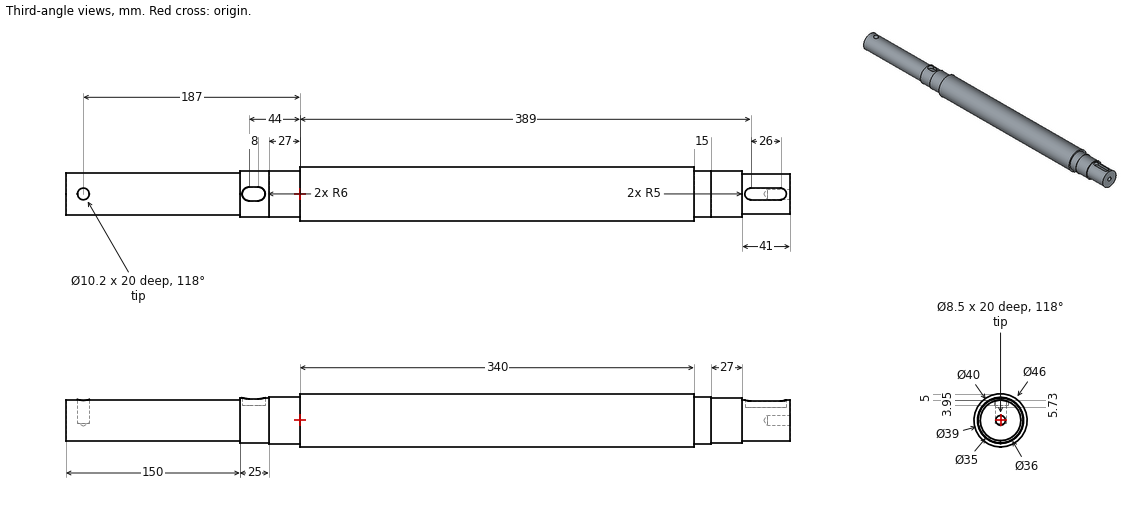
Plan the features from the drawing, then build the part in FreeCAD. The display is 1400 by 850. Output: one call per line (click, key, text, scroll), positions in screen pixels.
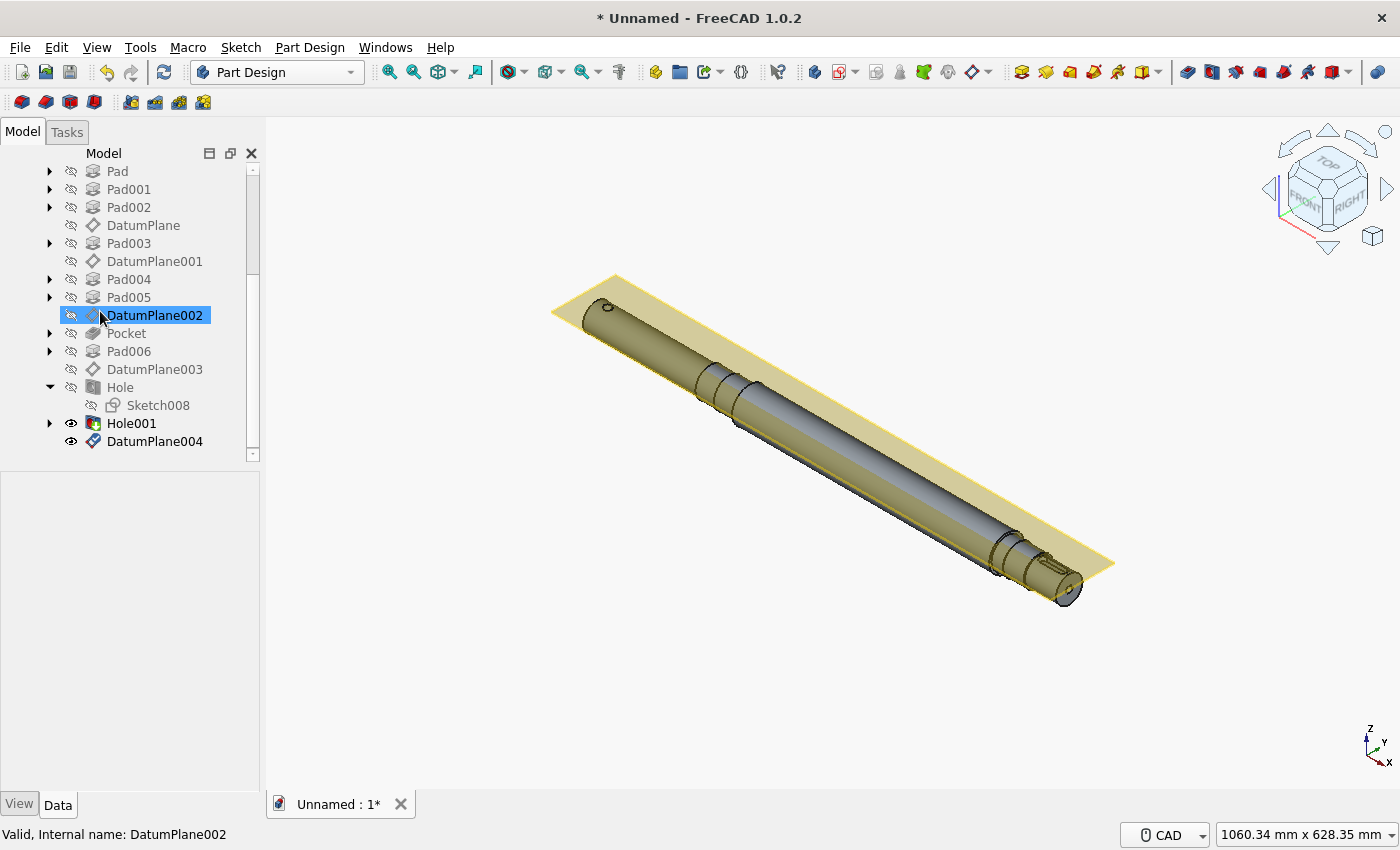
click(116, 441)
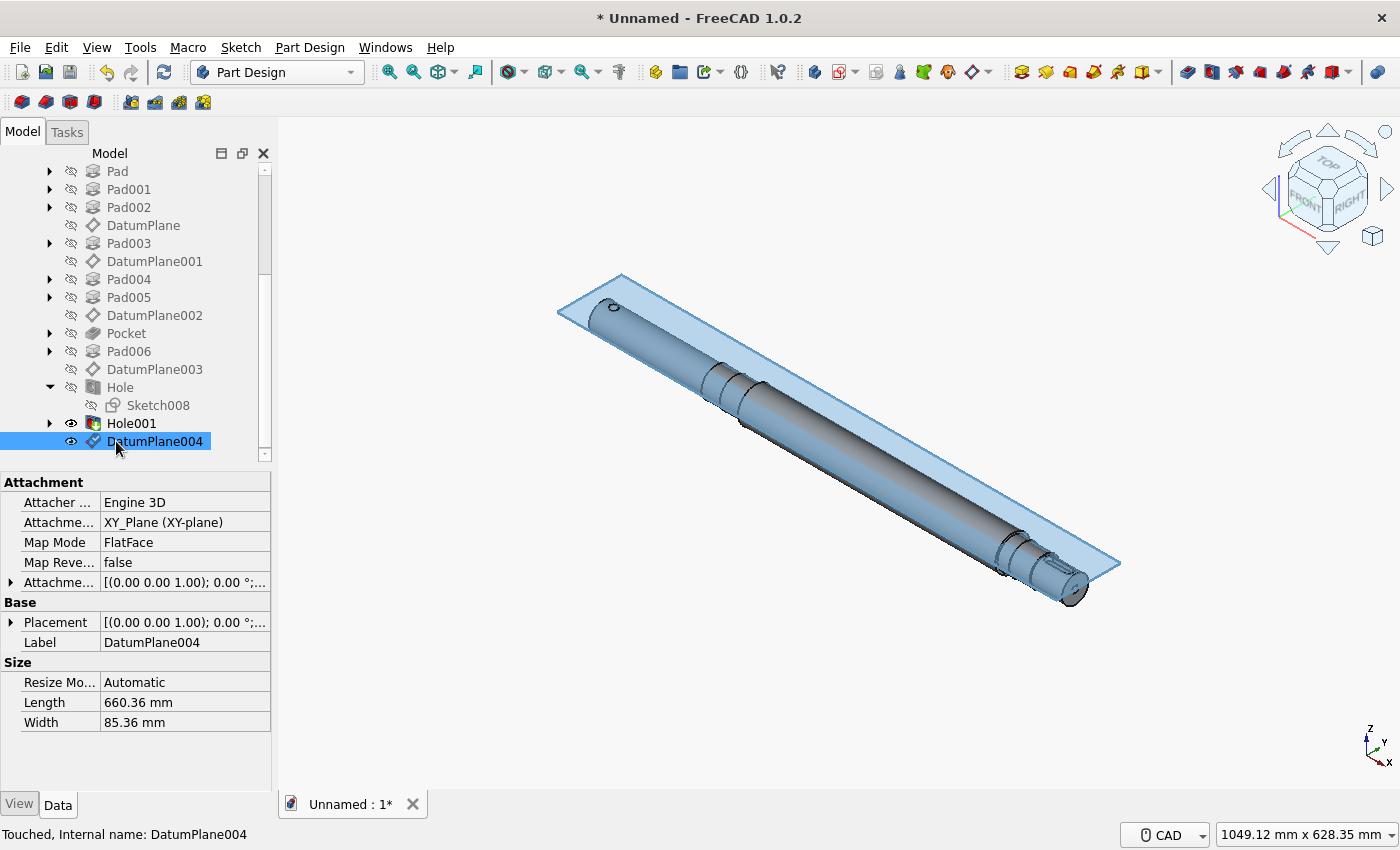
click(840, 72)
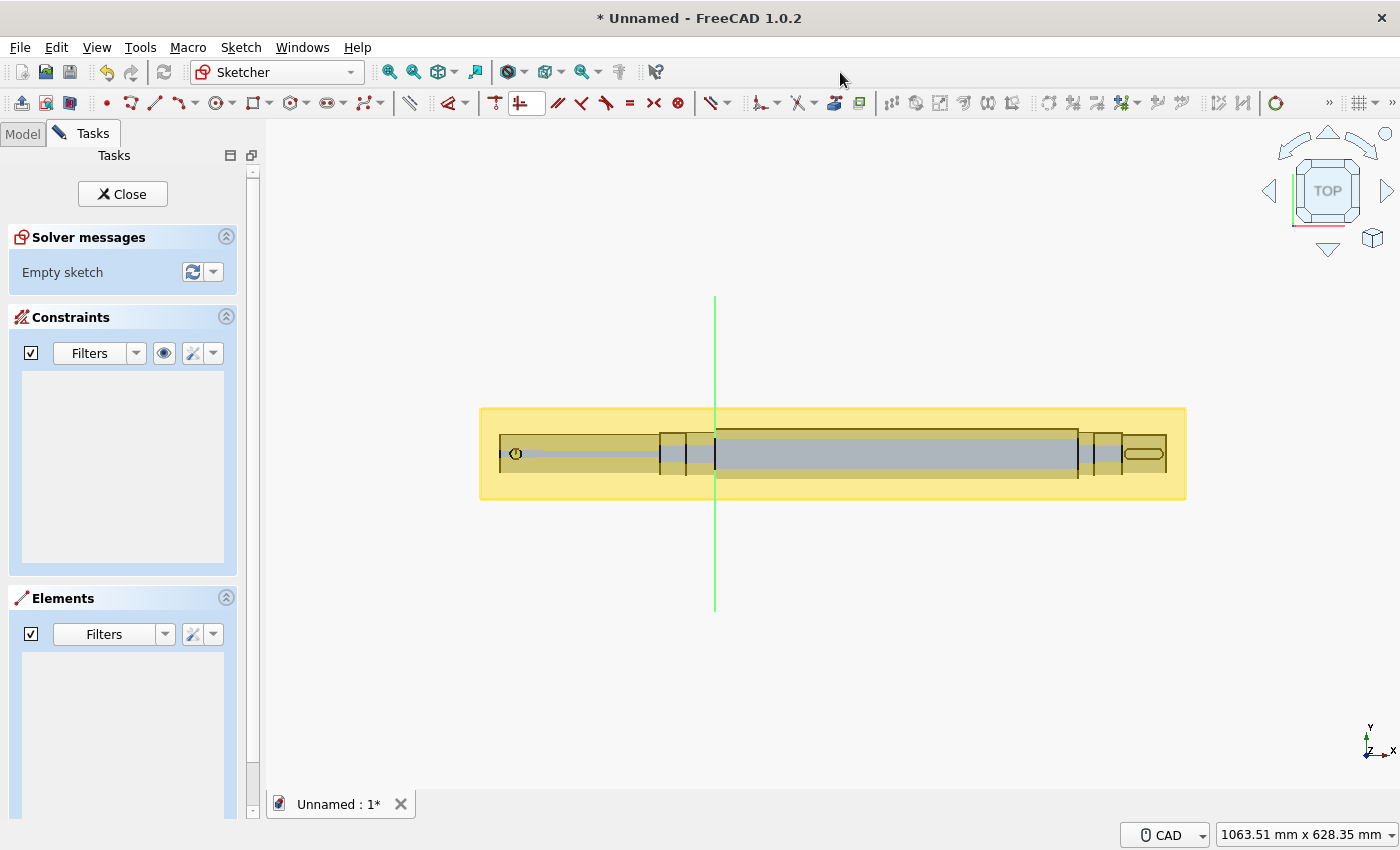
click(70, 104)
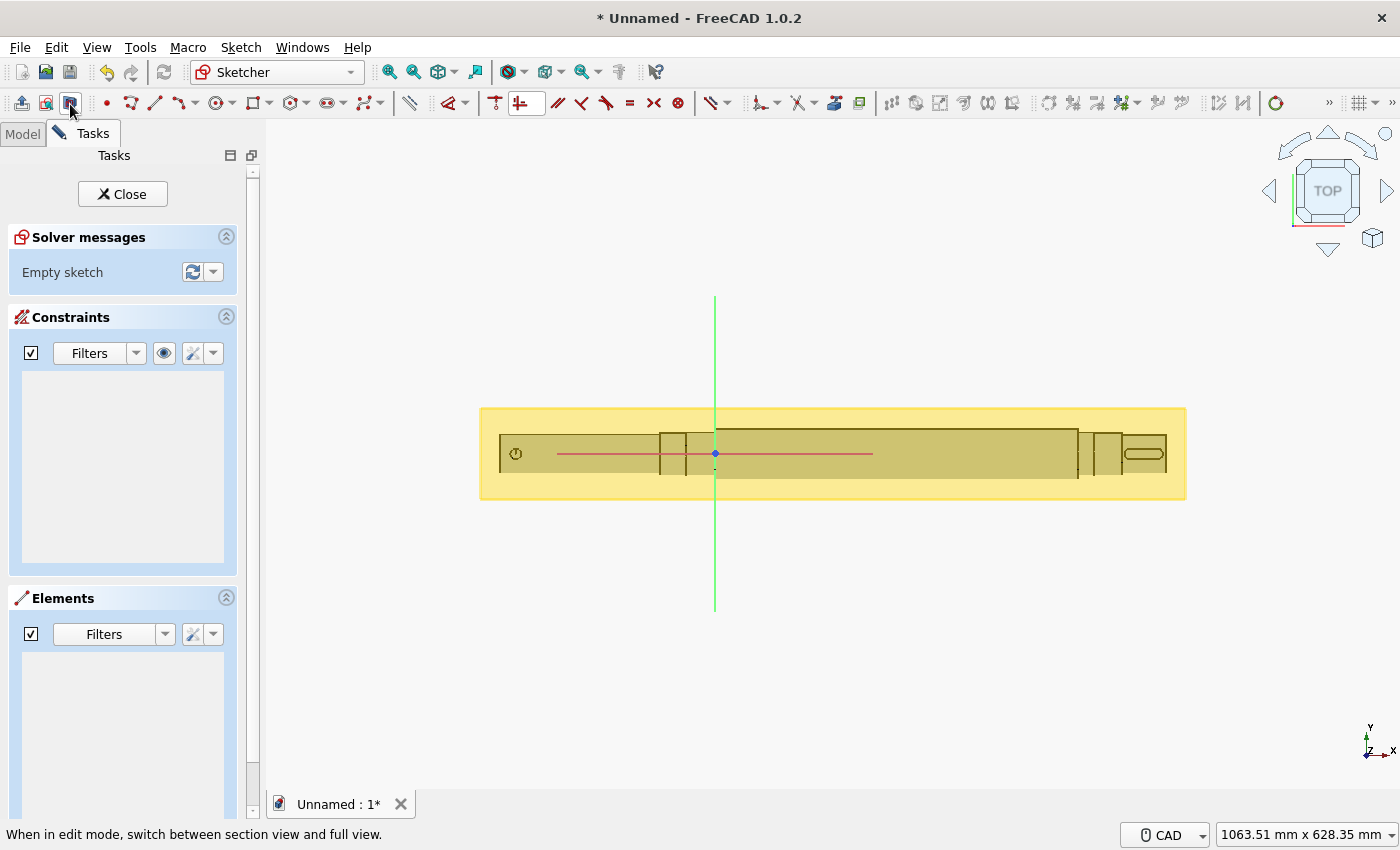
scroll(668, 454, up, 15)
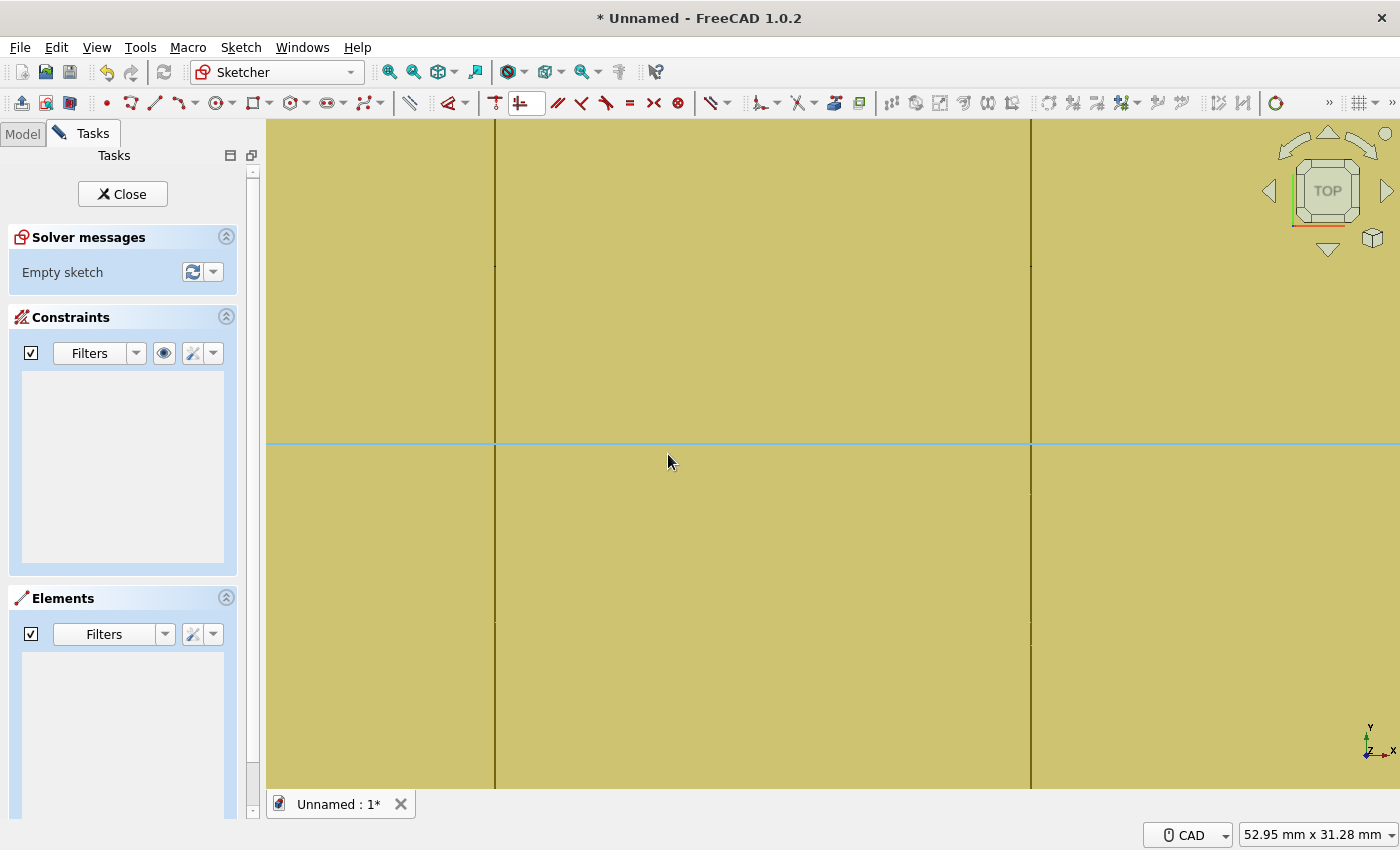
scroll(727, 425, up, 2)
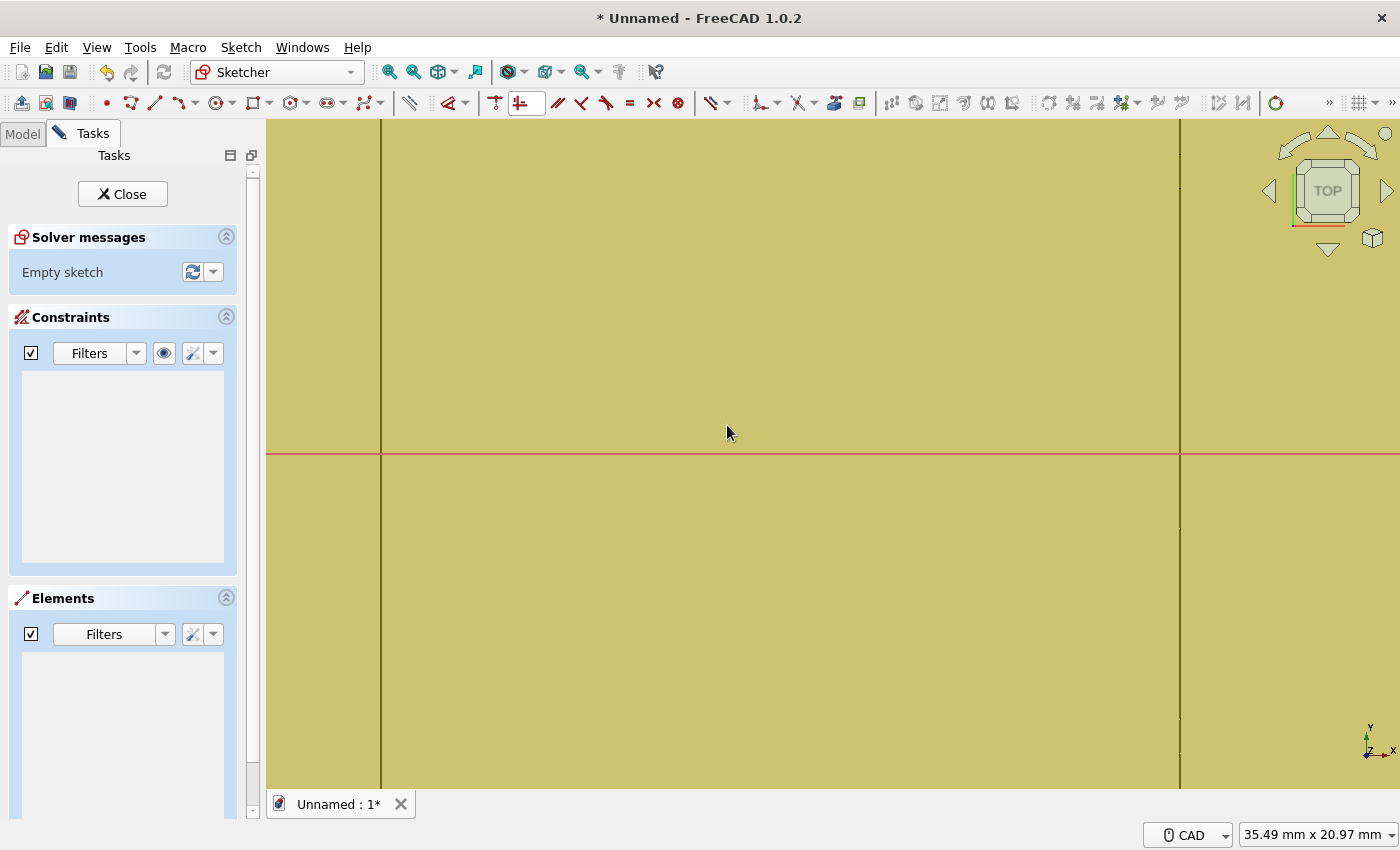
click(328, 104)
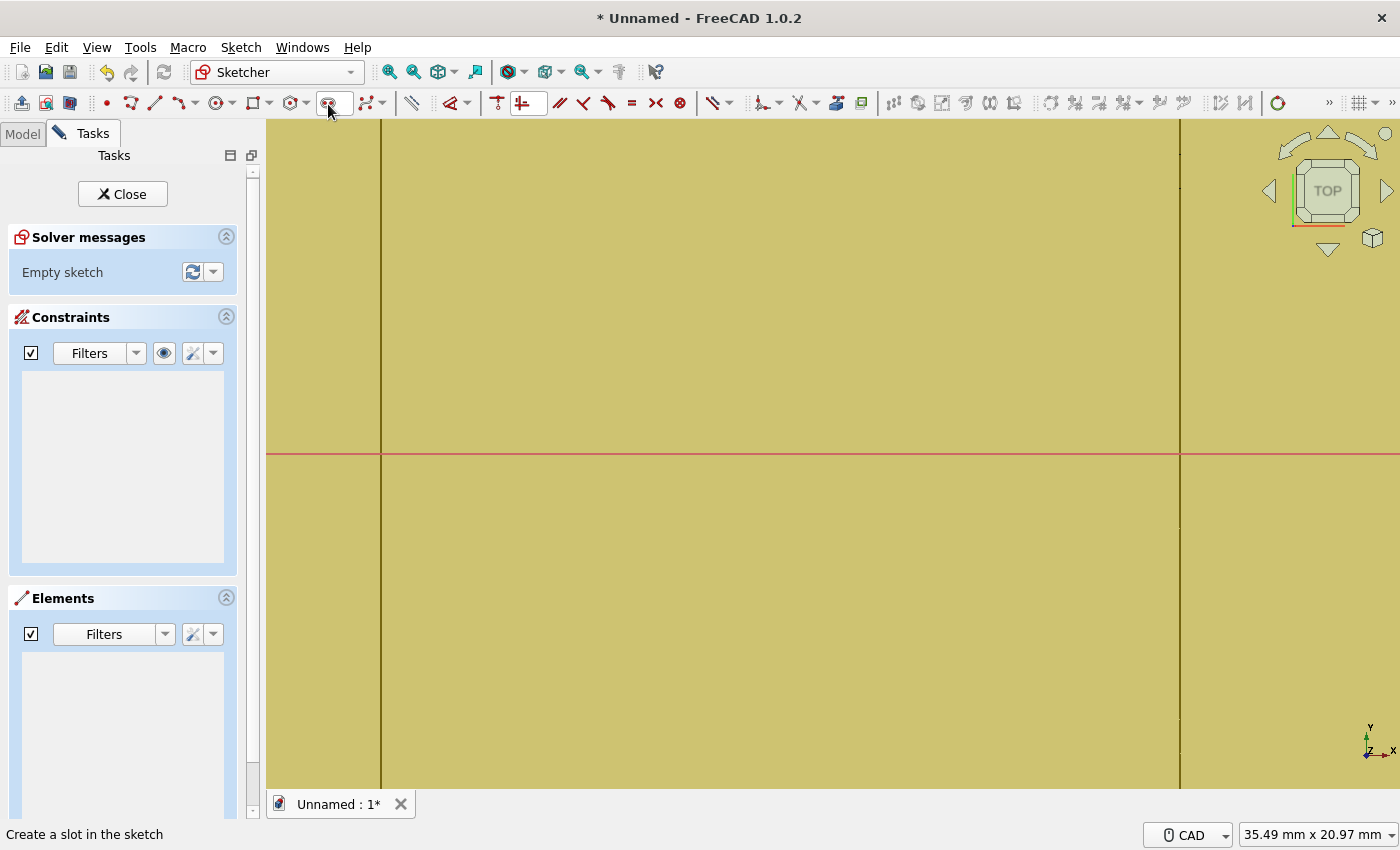
click(636, 454)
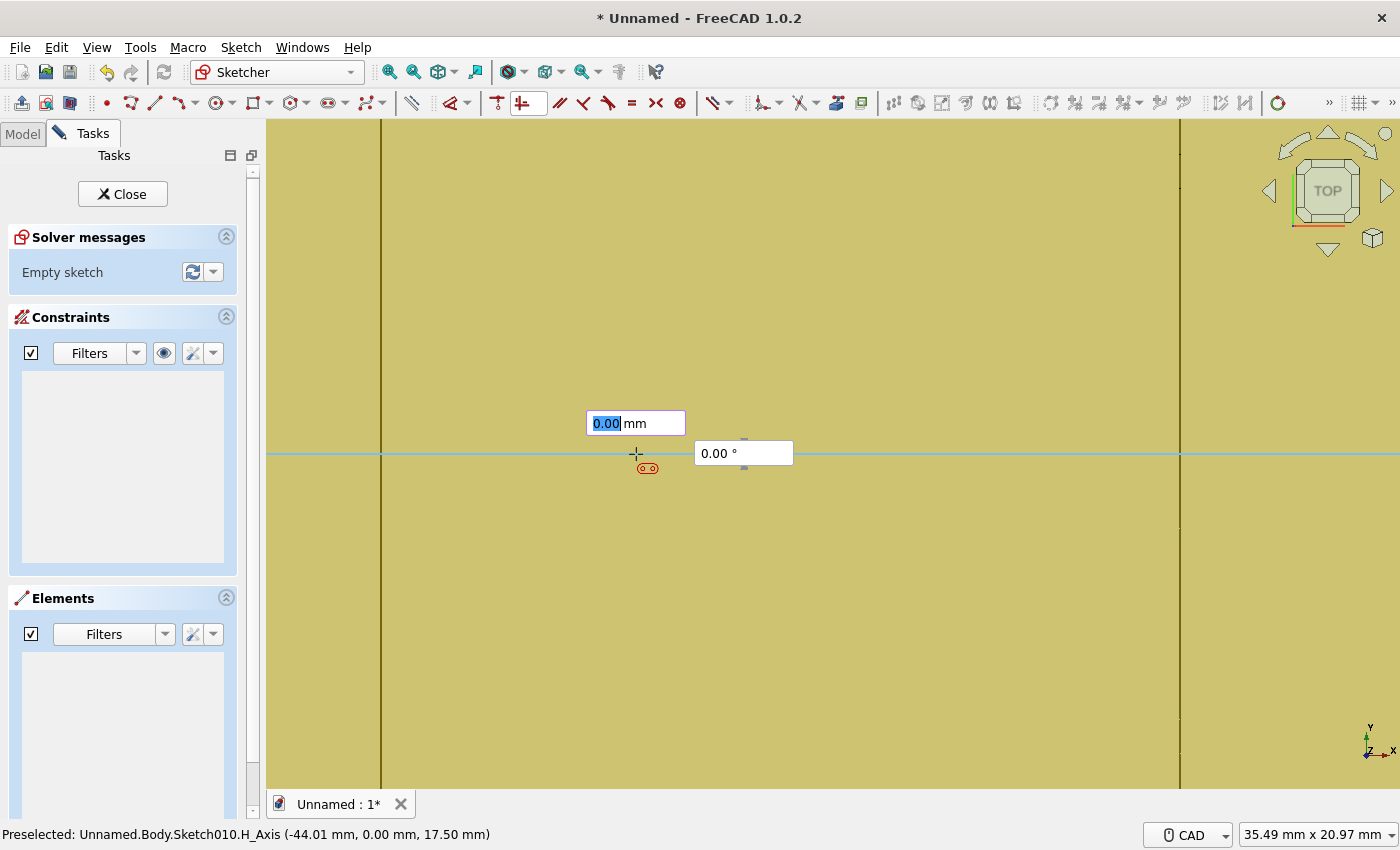
click(892, 445)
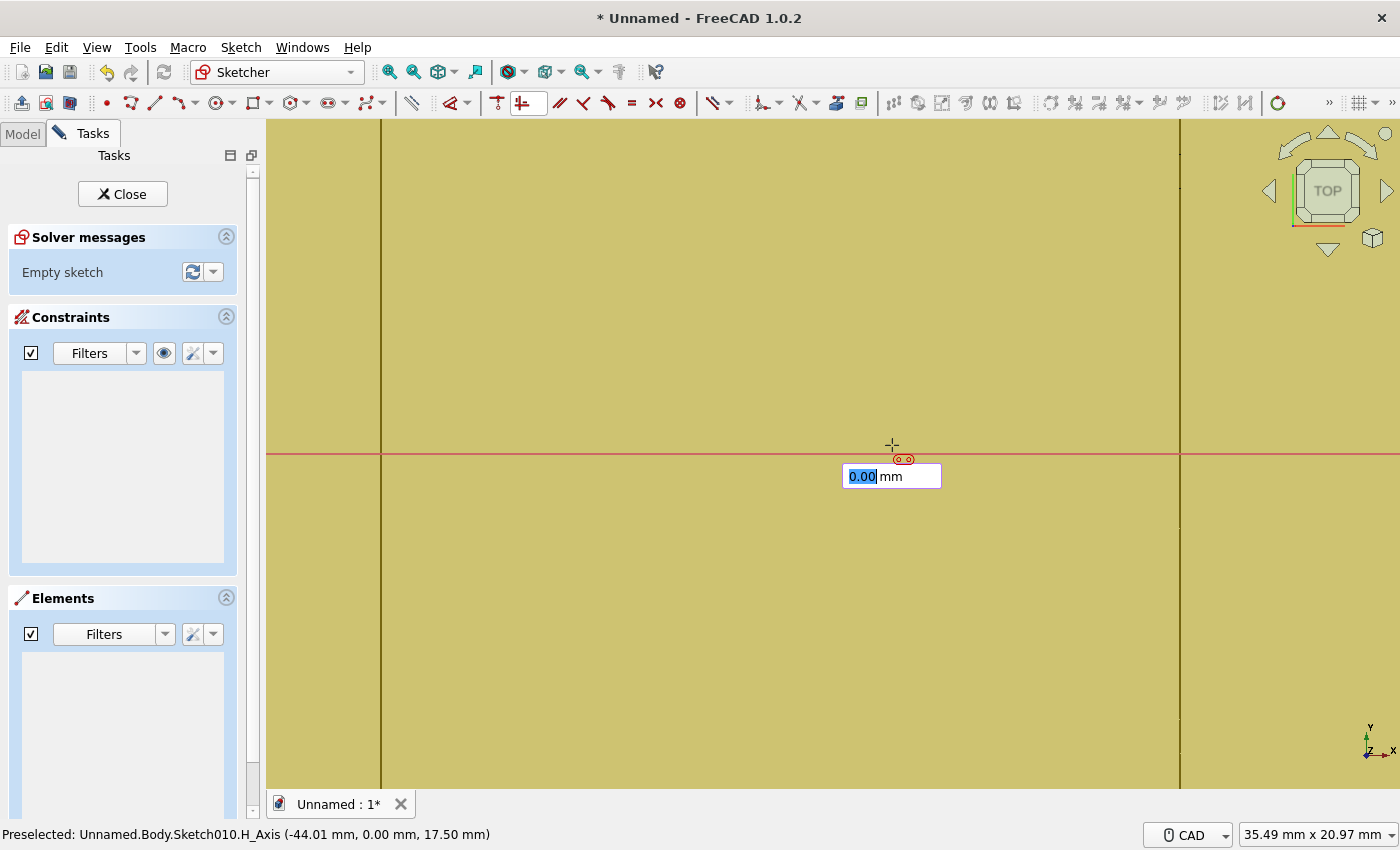
click(764, 645)
key(Escape)